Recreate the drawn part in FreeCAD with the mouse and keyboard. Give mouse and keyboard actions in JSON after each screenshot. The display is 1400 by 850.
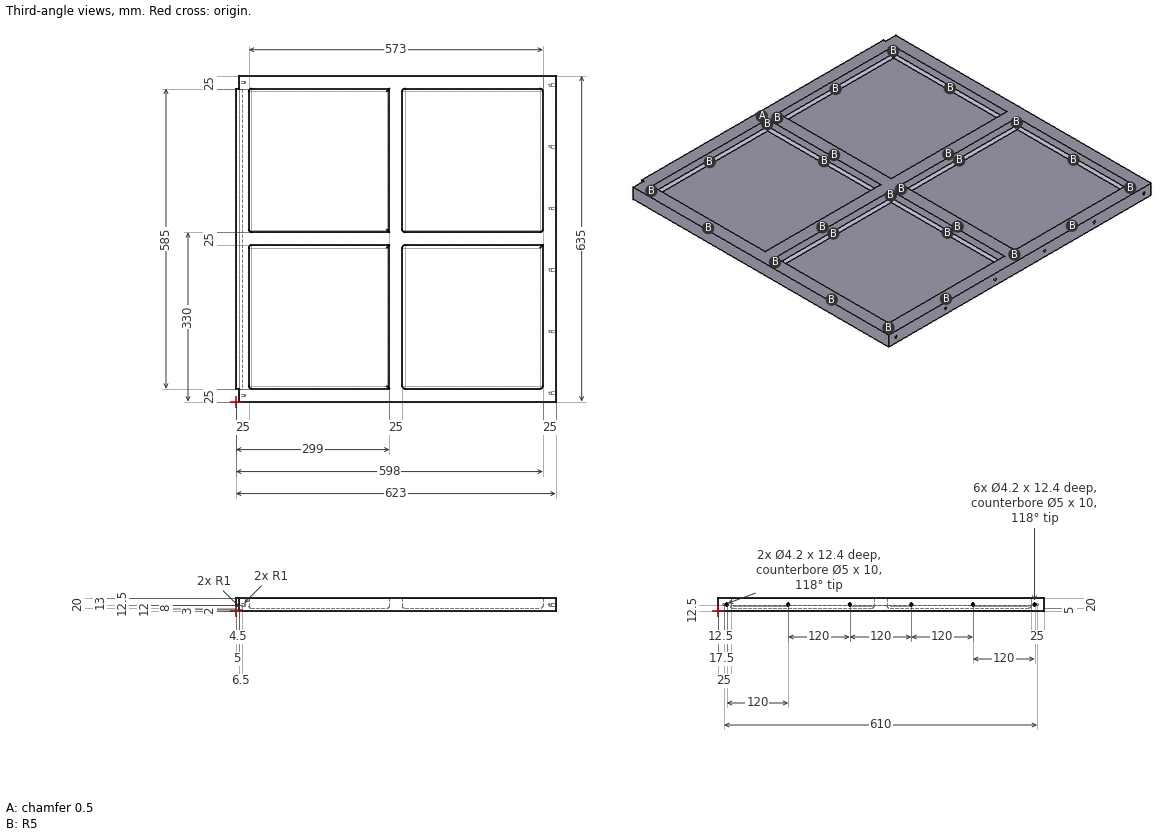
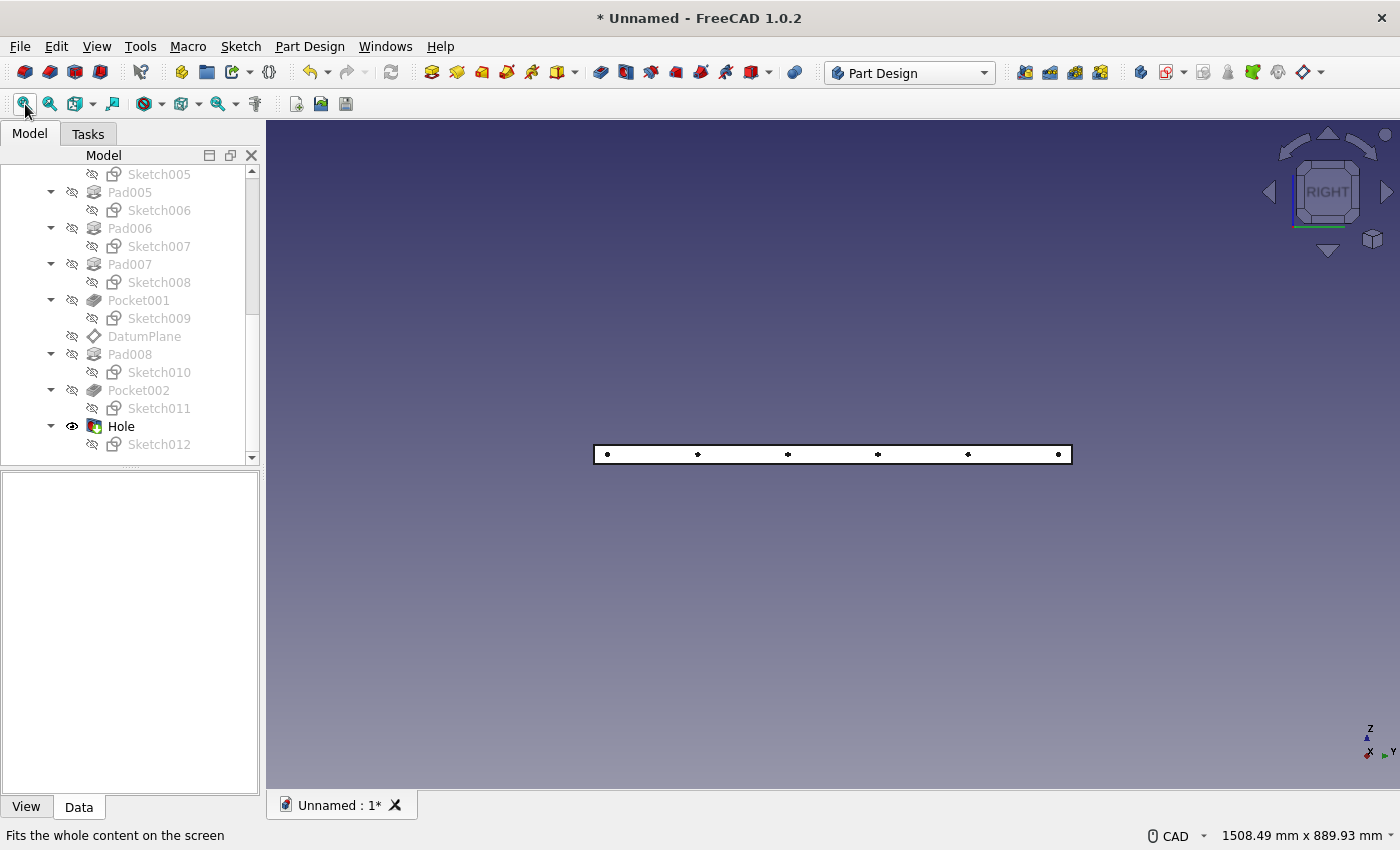
{"action": "key", "text": "6"}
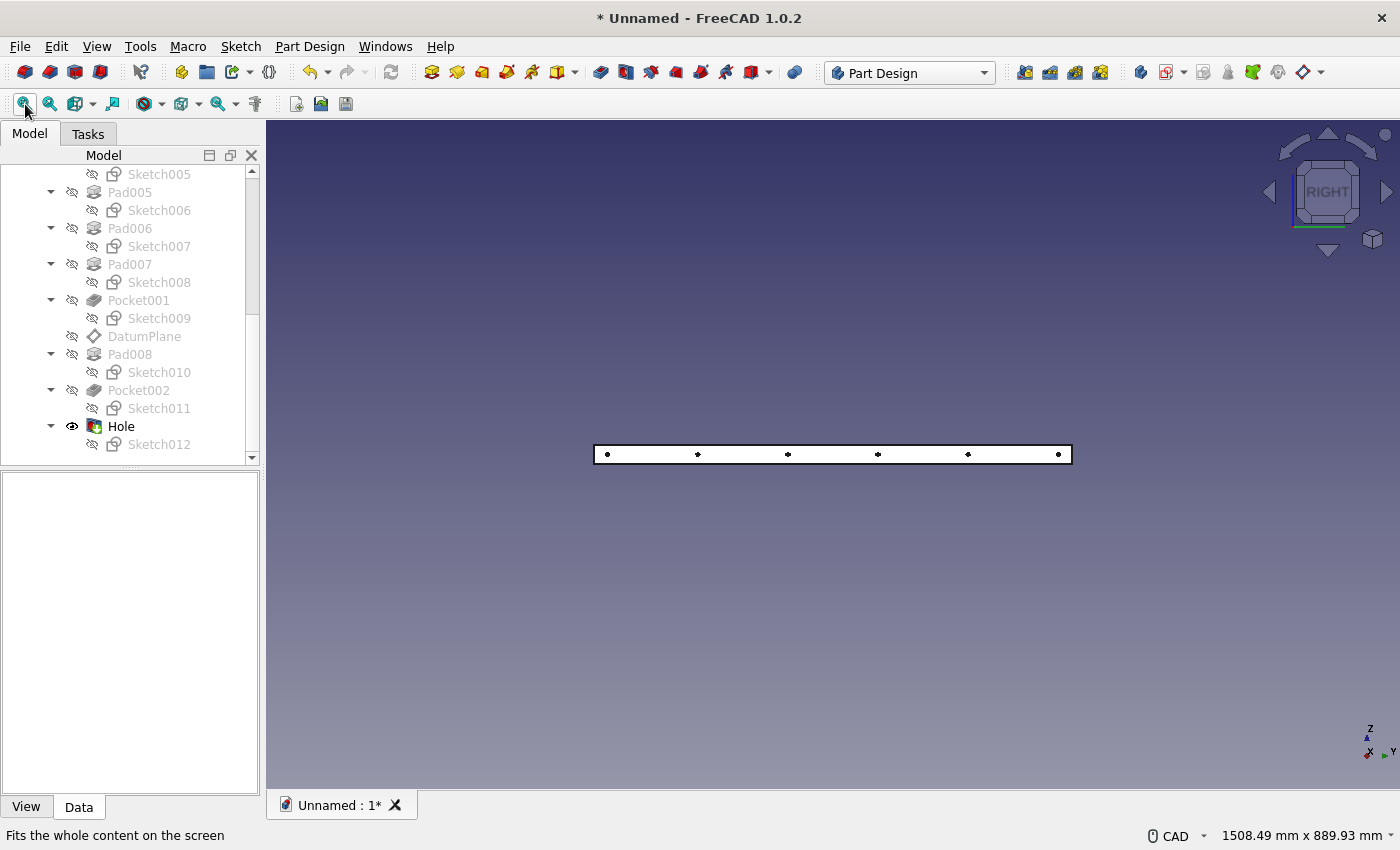
{"action": "left_click", "coordinate": [25, 104]}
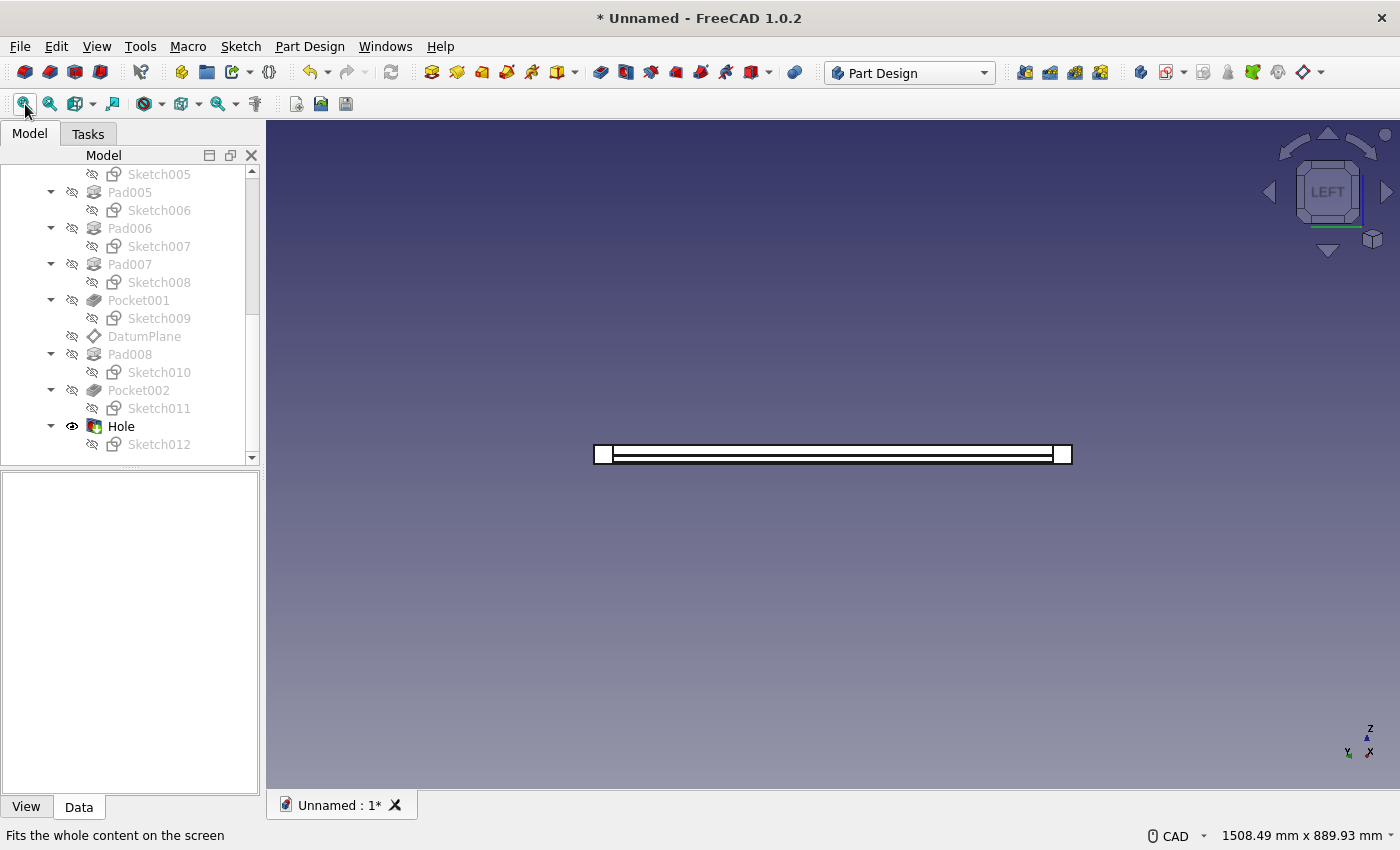
{"action": "scroll", "coordinate": [1038, 462], "scroll_direction": "up", "scroll_amount": 15}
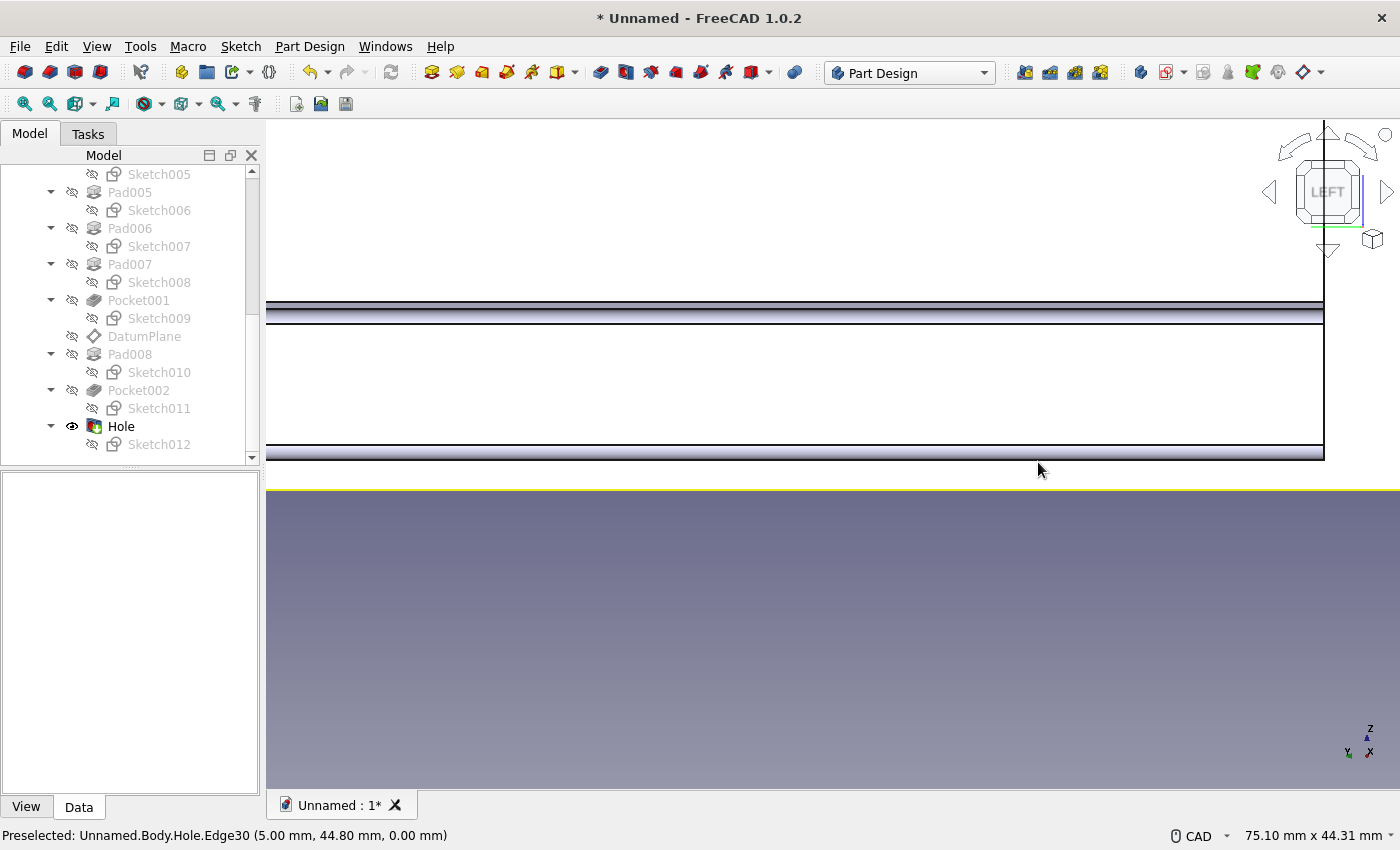
{"action": "scroll", "coordinate": [1017, 462], "scroll_direction": "up", "scroll_amount": 7}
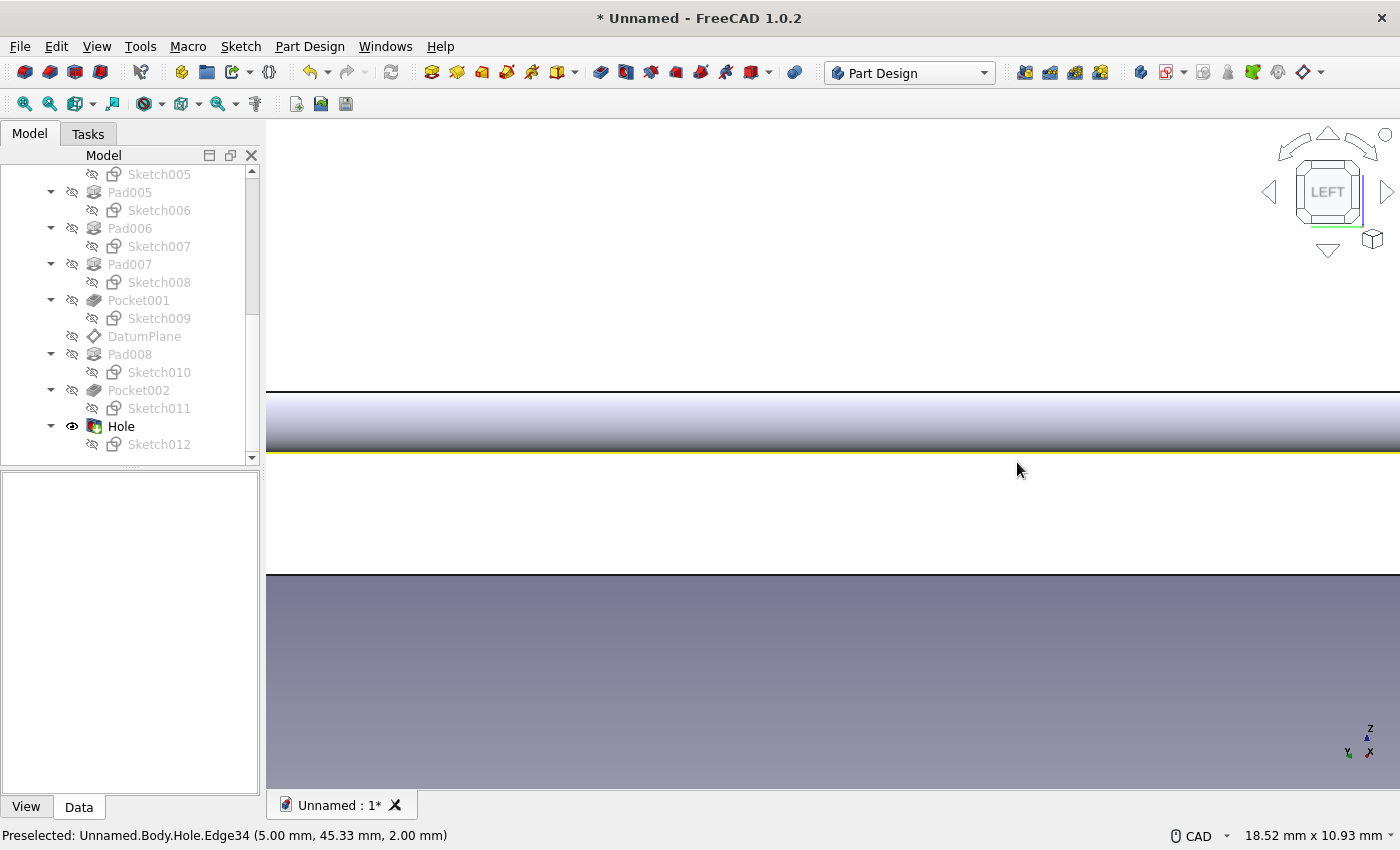
{"action": "left_click", "coordinate": [1013, 465]}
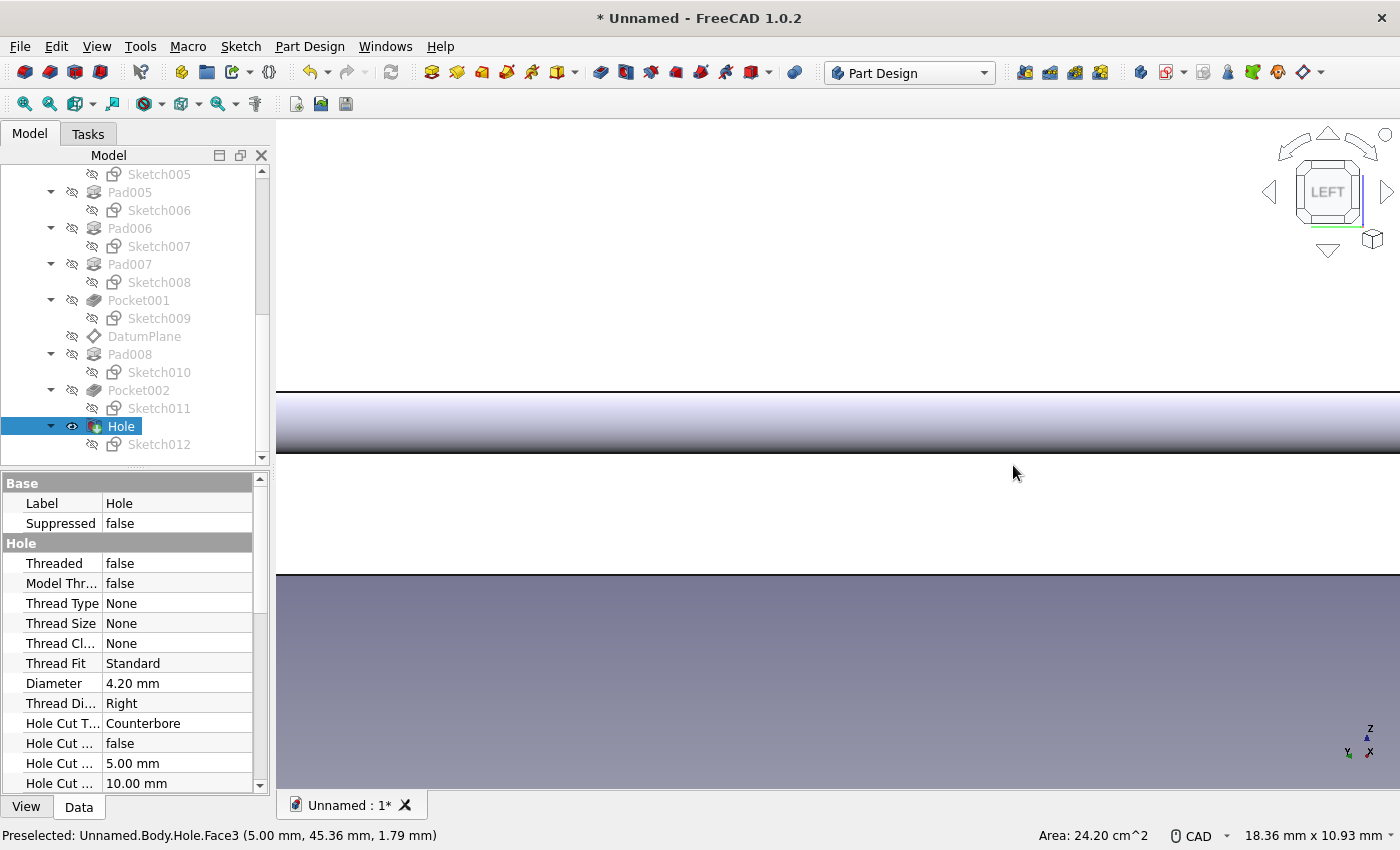
{"action": "left_click", "coordinate": [1166, 72]}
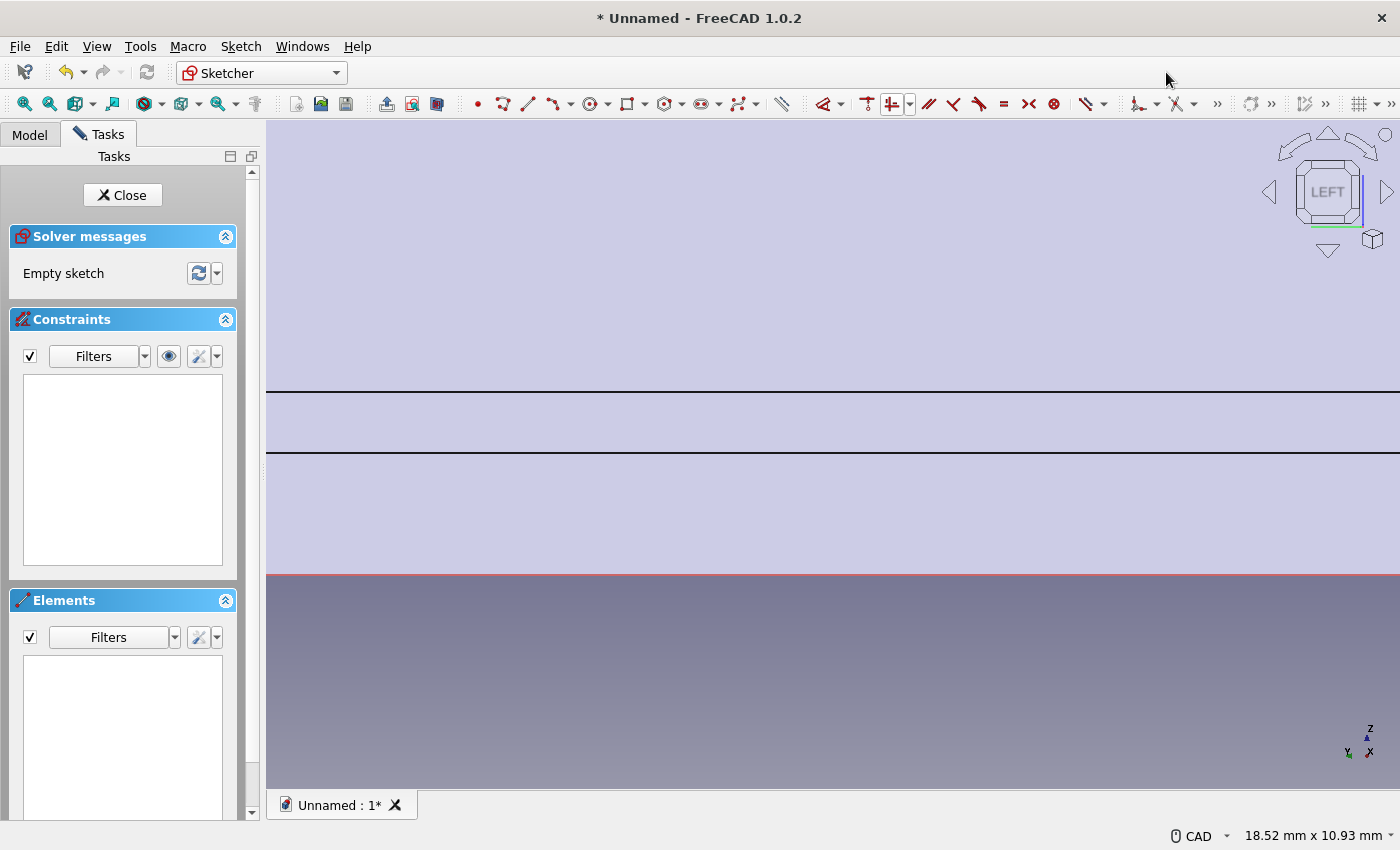
{"action": "left_click", "coordinate": [437, 104]}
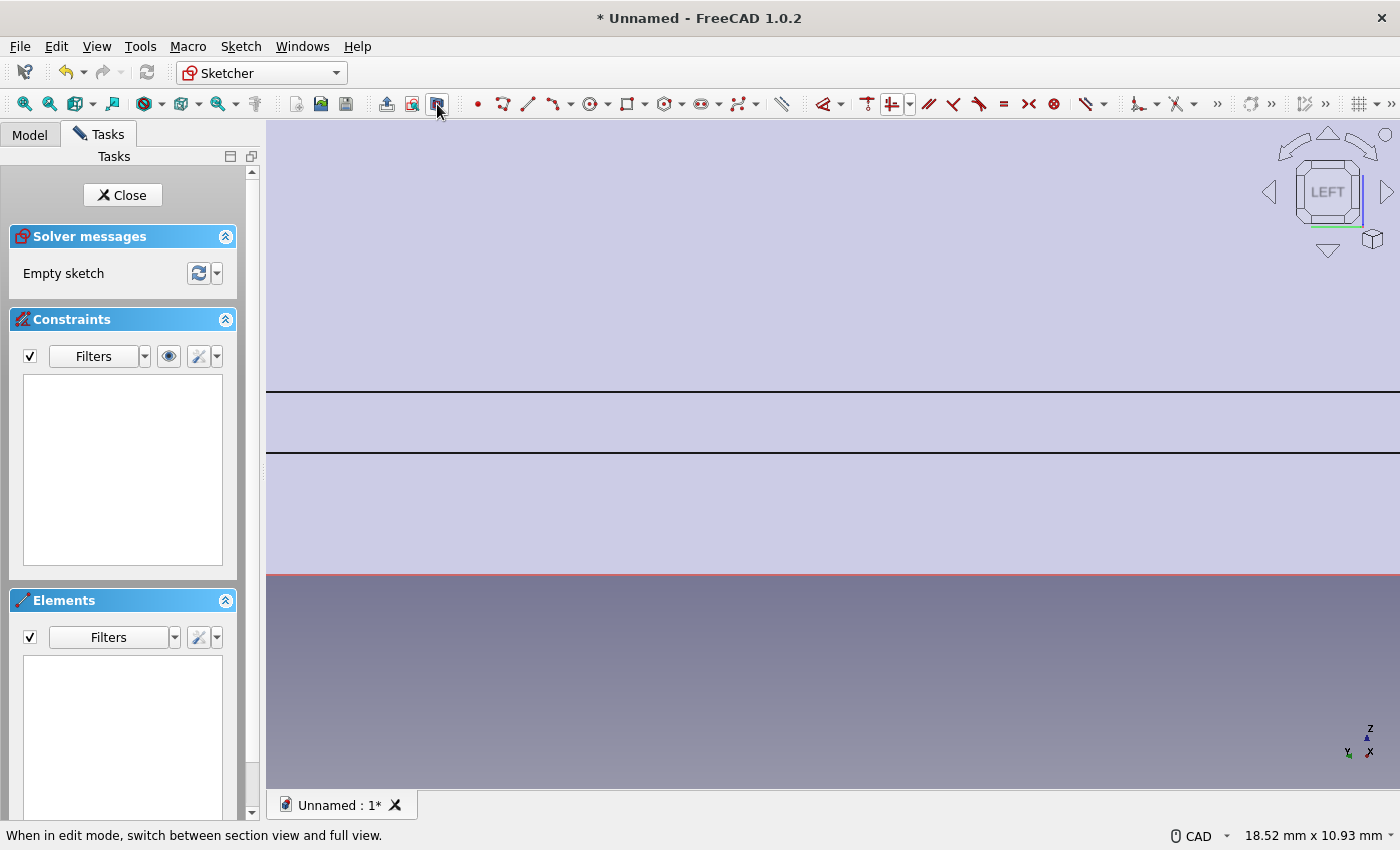
{"action": "scroll", "coordinate": [764, 454], "scroll_direction": "down", "scroll_amount": 15}